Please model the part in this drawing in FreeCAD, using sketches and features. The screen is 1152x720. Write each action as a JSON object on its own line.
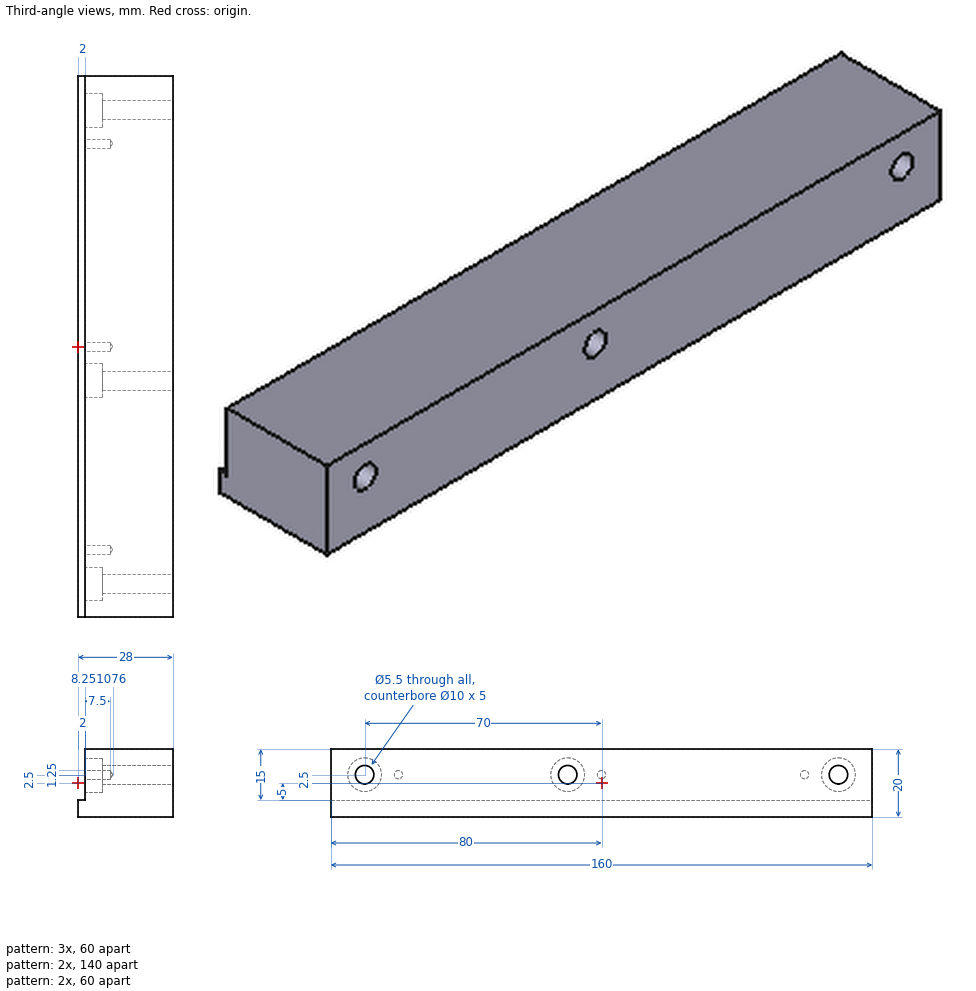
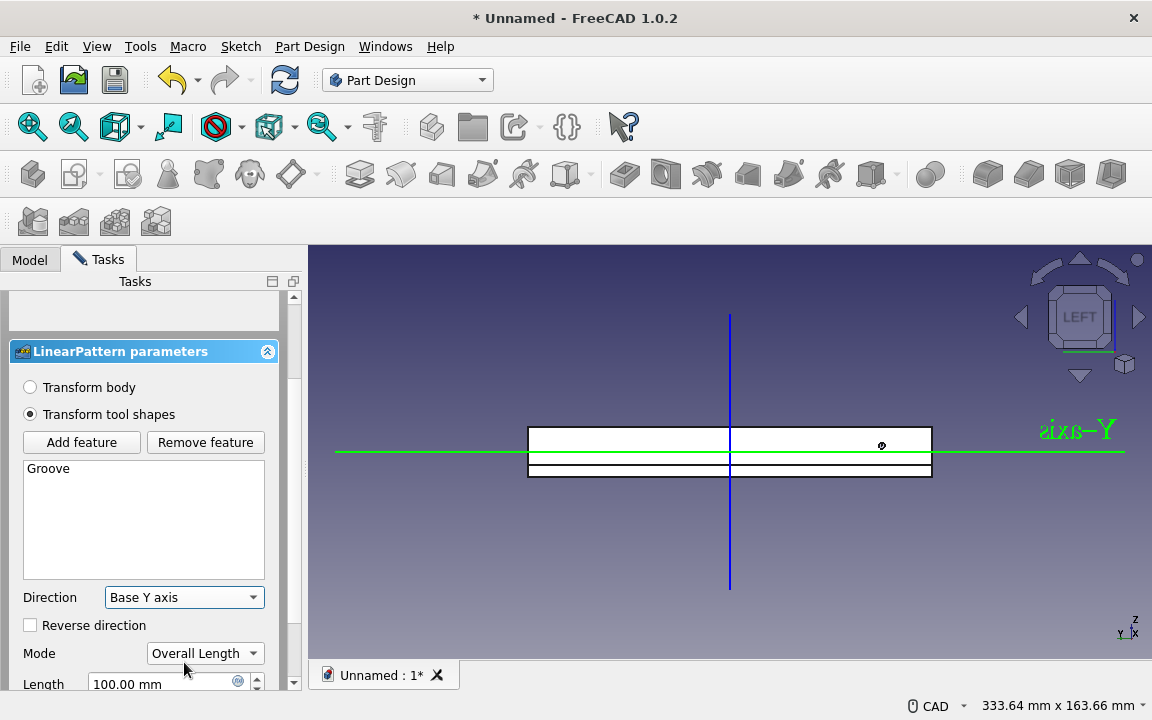
{"action": "left_click", "coordinate": [206, 654]}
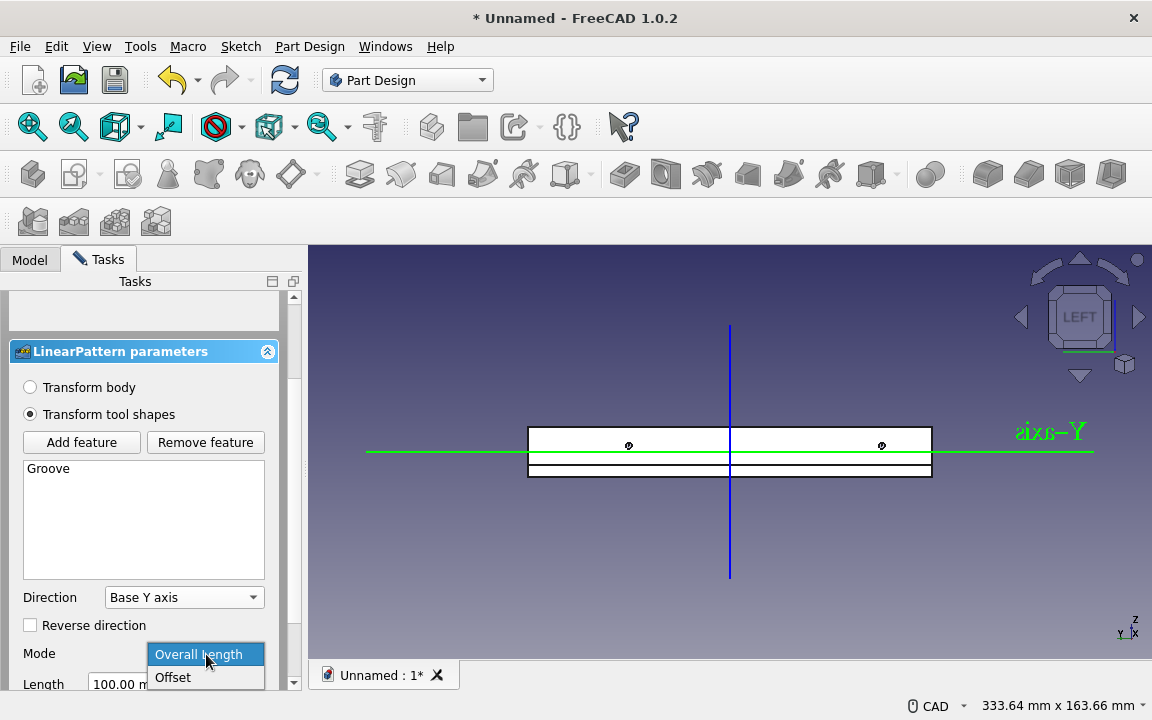
{"action": "left_click", "coordinate": [204, 678]}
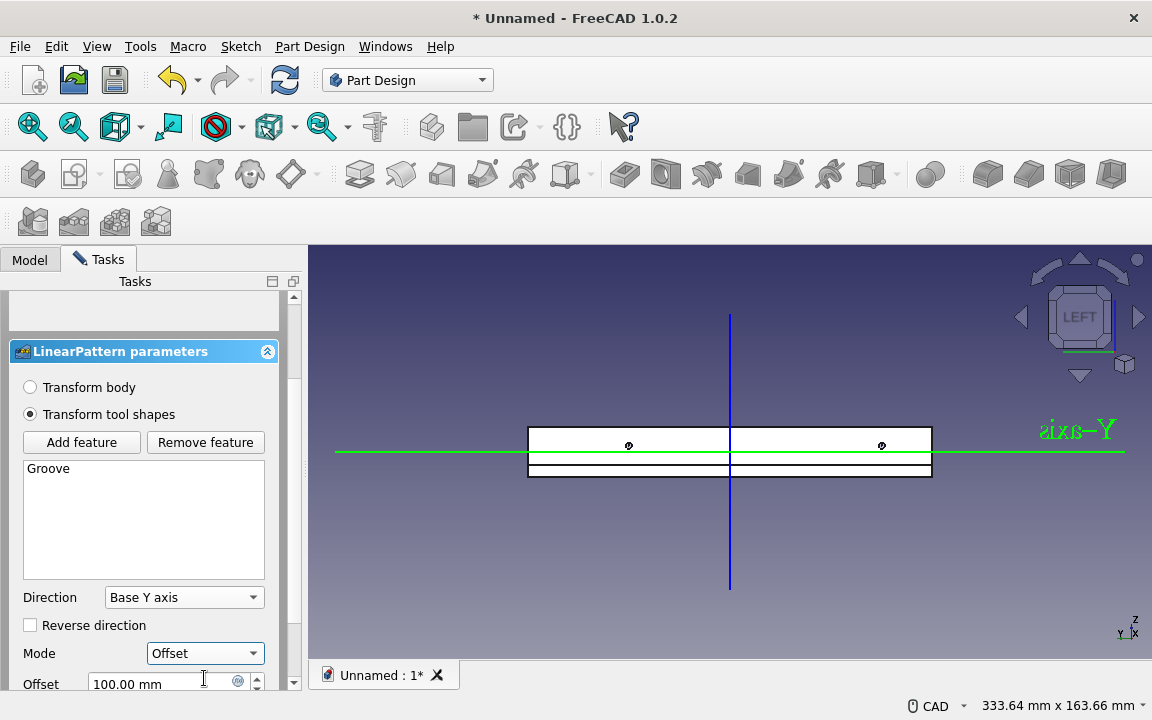
{"action": "scroll", "coordinate": [294, 490], "scroll_direction": "down", "scroll_amount": 2}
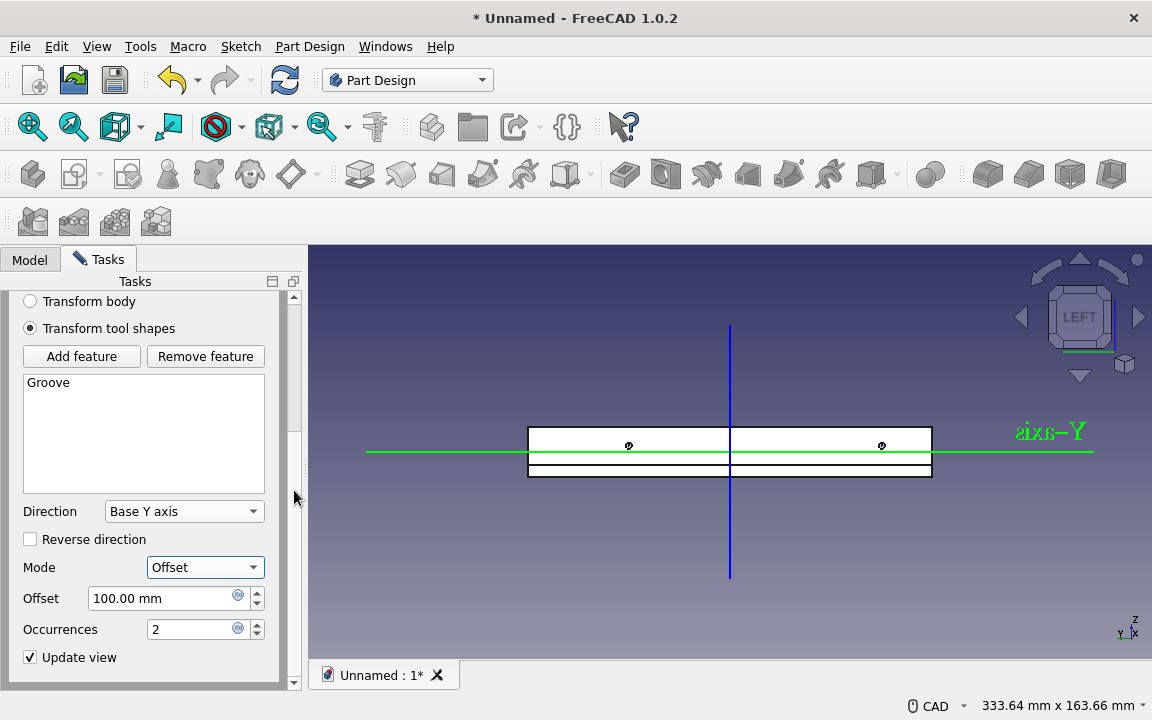
{"action": "triple_click", "coordinate": [170, 598]}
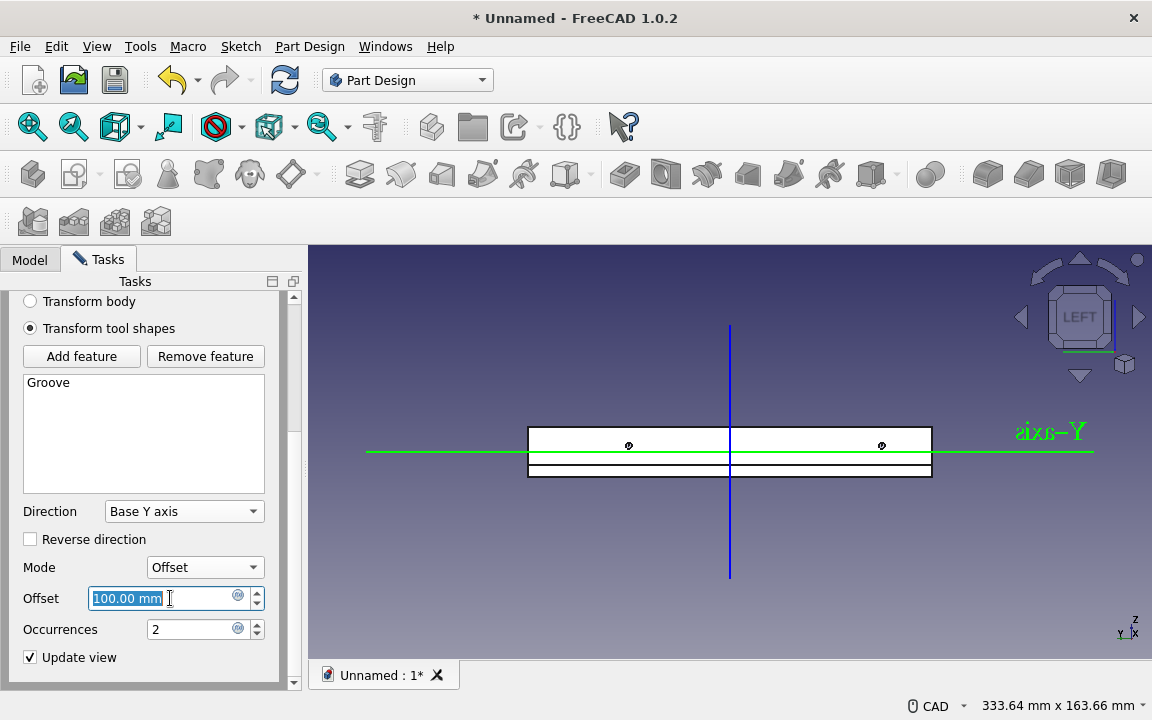
{"action": "type", "text": "60"}
{"action": "key", "text": "Tab"}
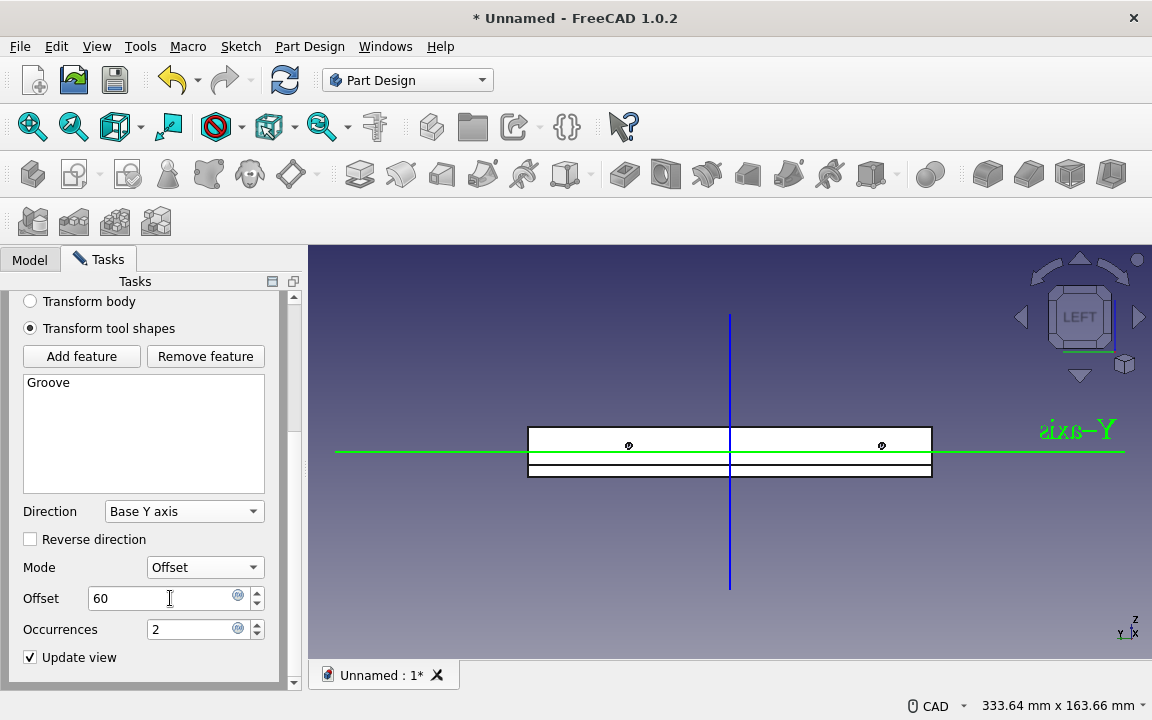
{"action": "triple_click", "coordinate": [199, 630]}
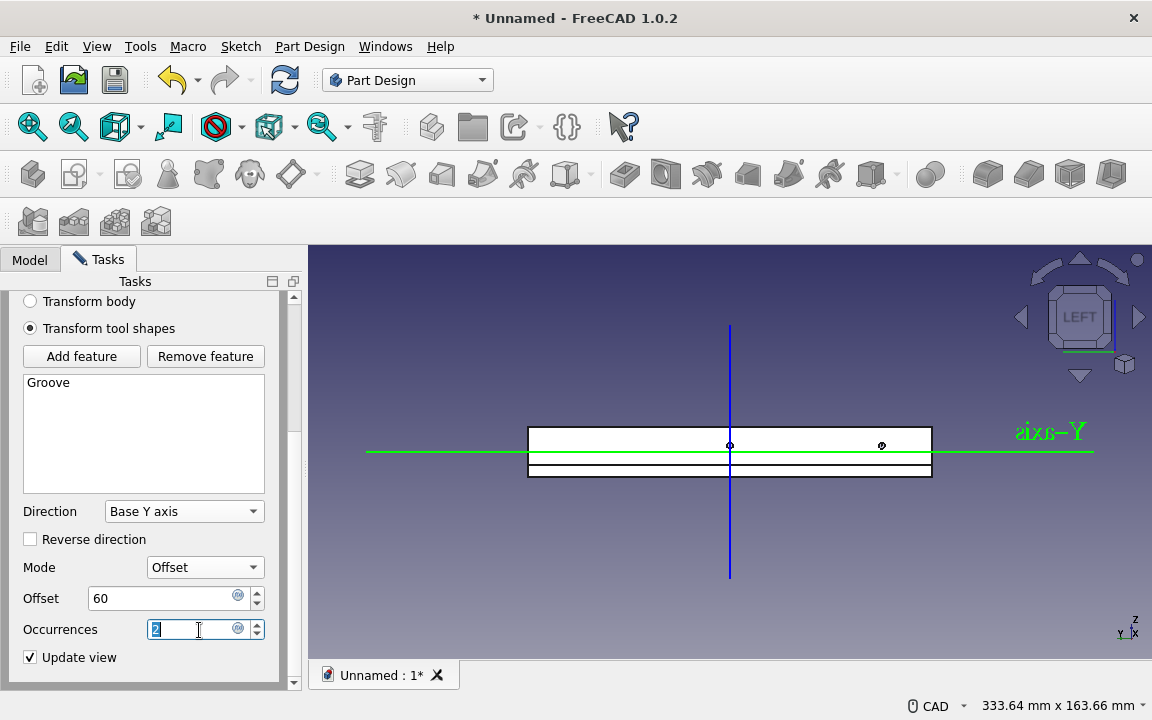
{"action": "type", "text": "3"}
{"action": "key", "text": "Tab"}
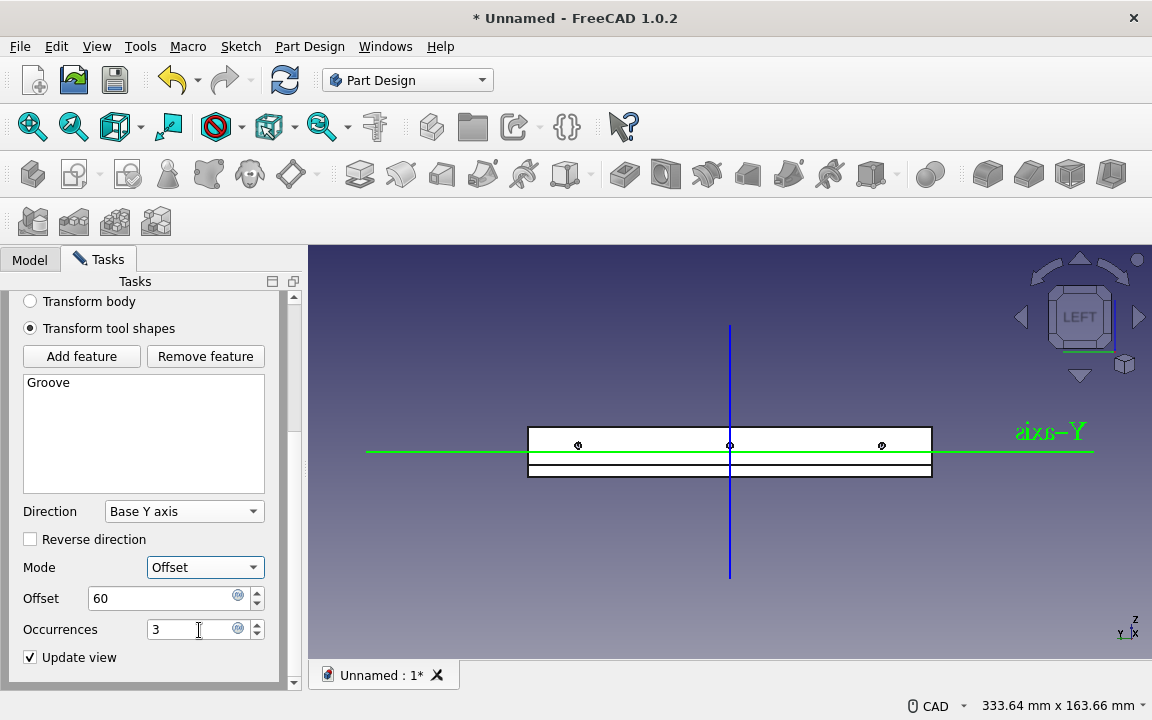
{"action": "scroll", "coordinate": [294, 490], "scroll_direction": "up", "scroll_amount": 5}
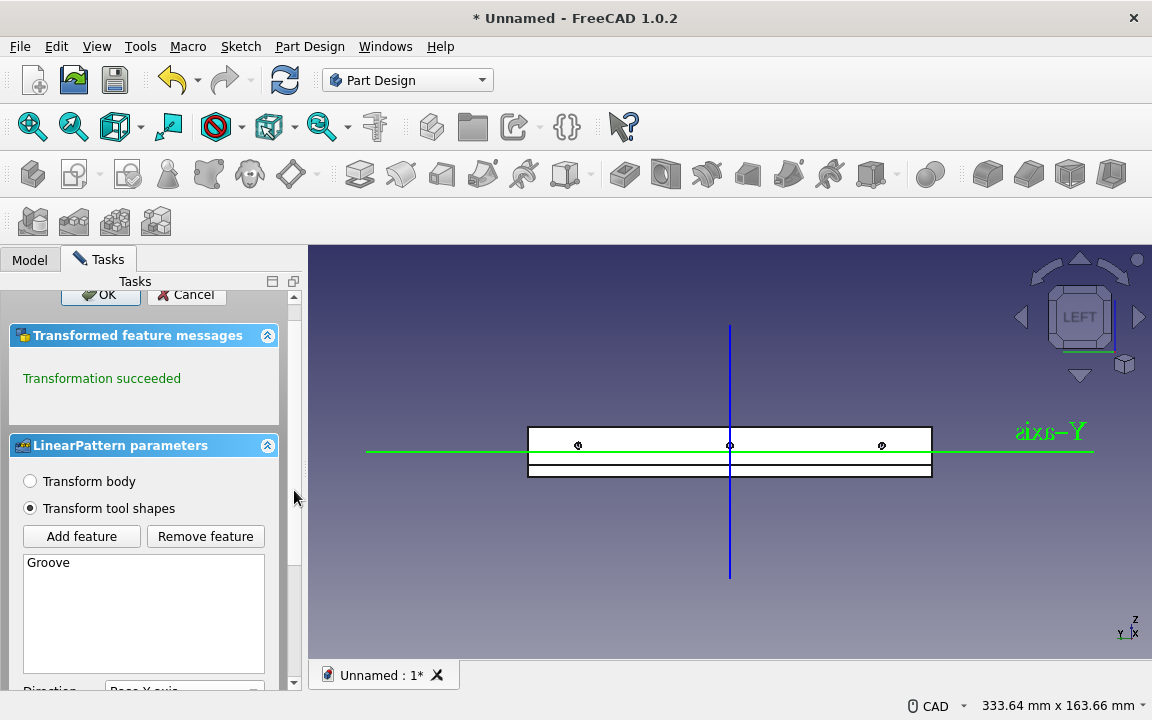
{"action": "left_click", "coordinate": [101, 320]}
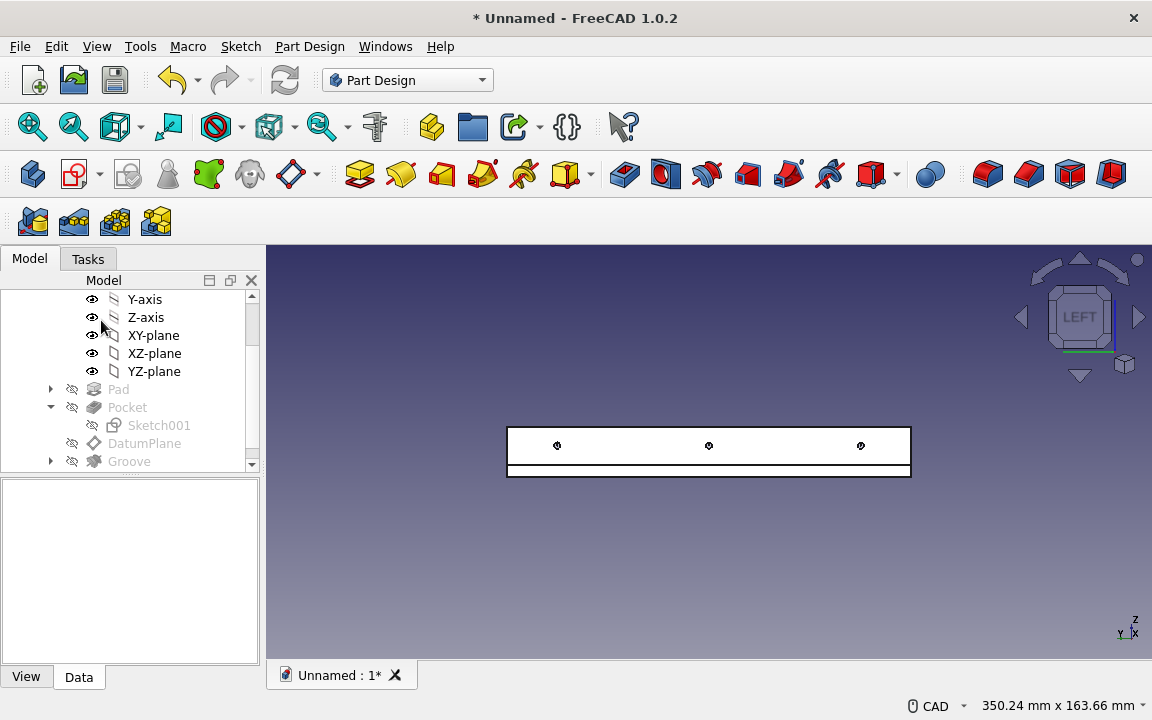
{"action": "left_click", "coordinate": [593, 445]}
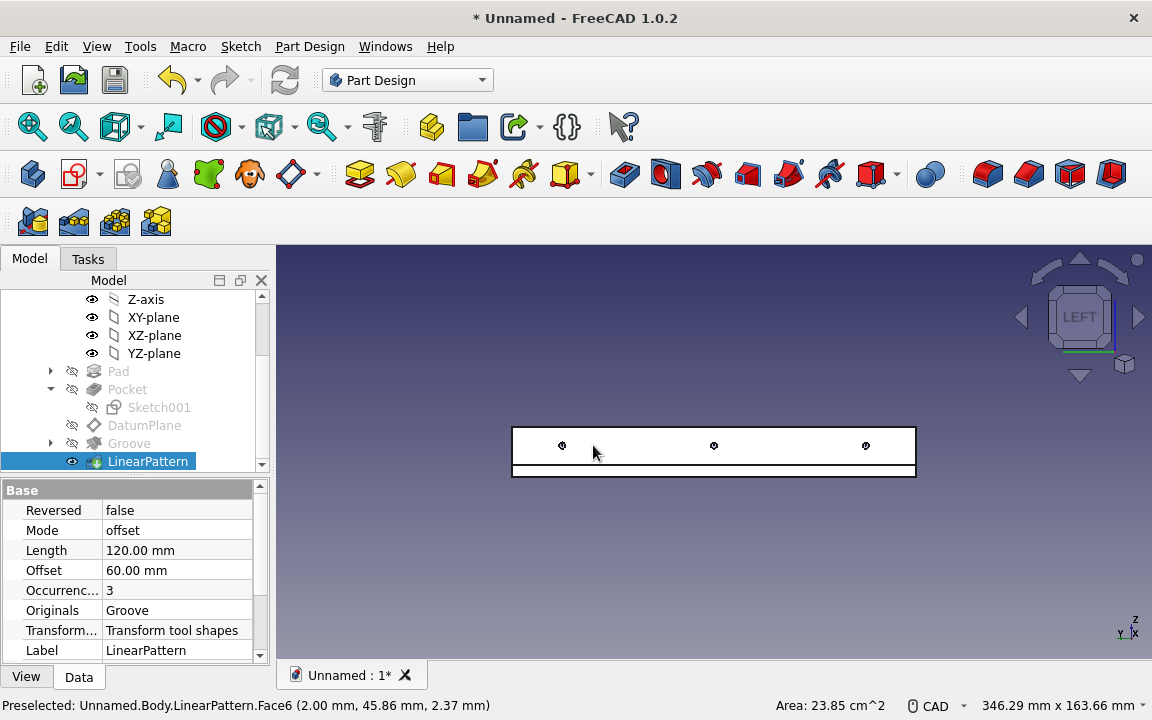
{"action": "left_click", "coordinate": [74, 174]}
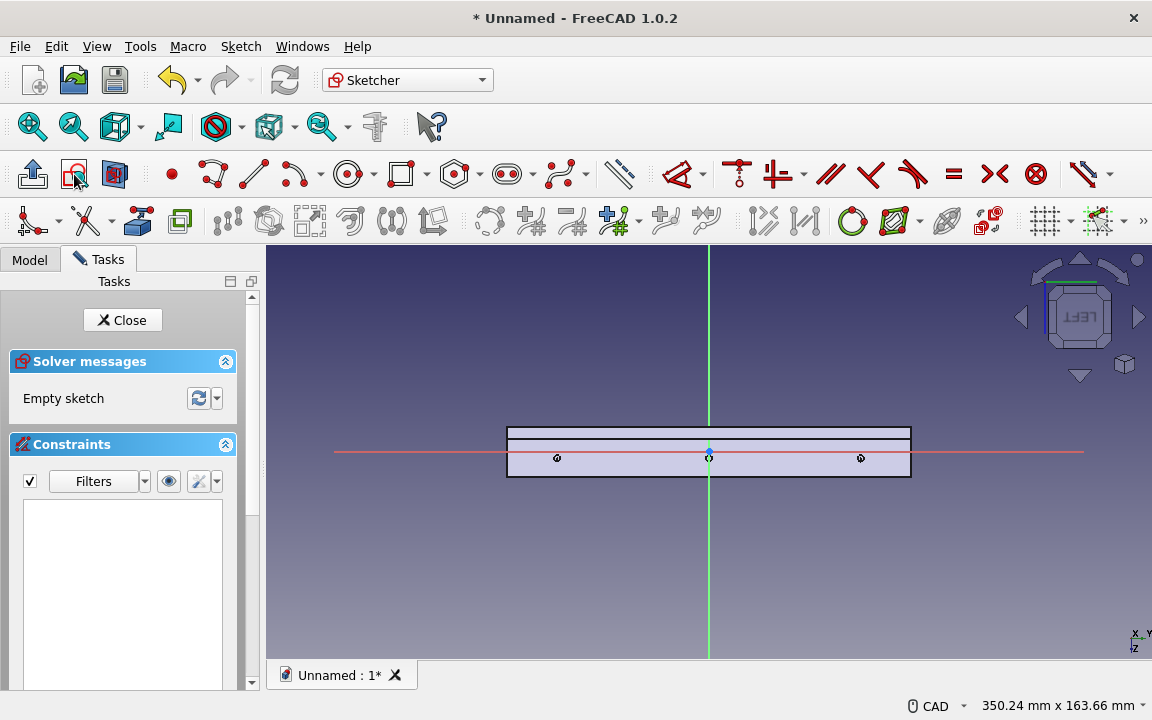
{"action": "scroll", "coordinate": [525, 459], "scroll_direction": "up", "scroll_amount": 14}